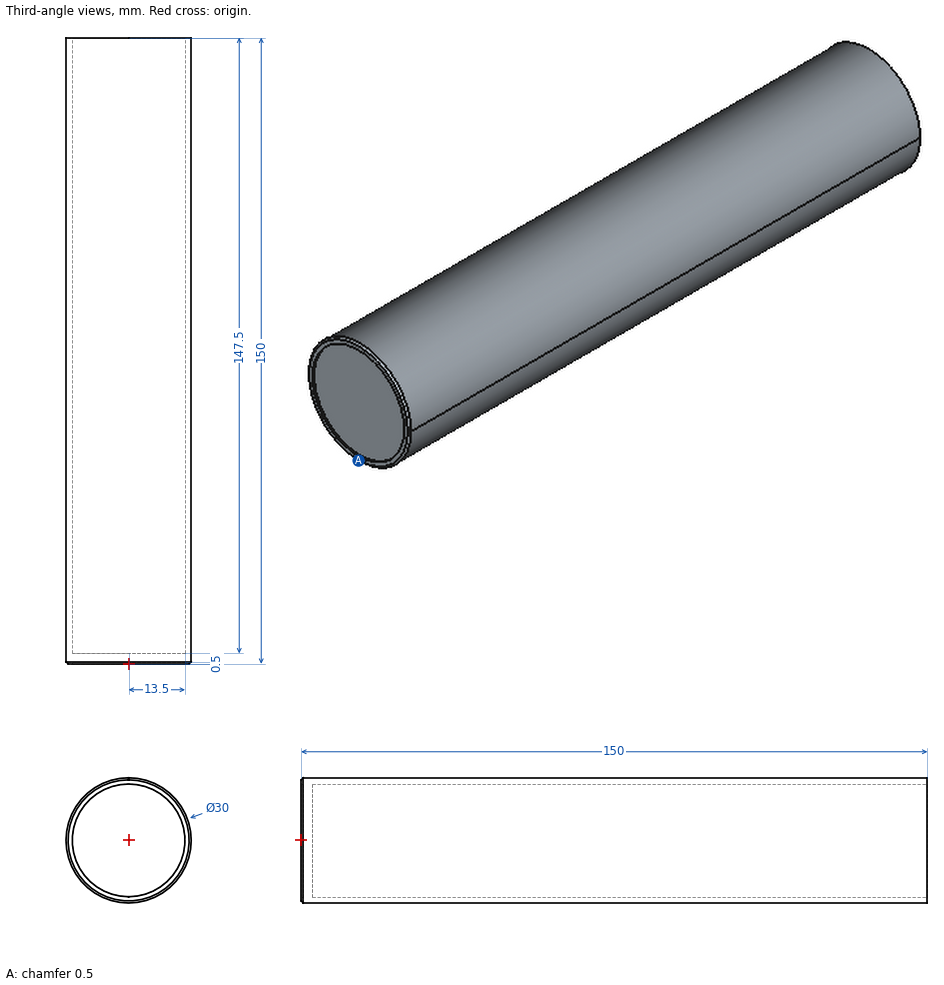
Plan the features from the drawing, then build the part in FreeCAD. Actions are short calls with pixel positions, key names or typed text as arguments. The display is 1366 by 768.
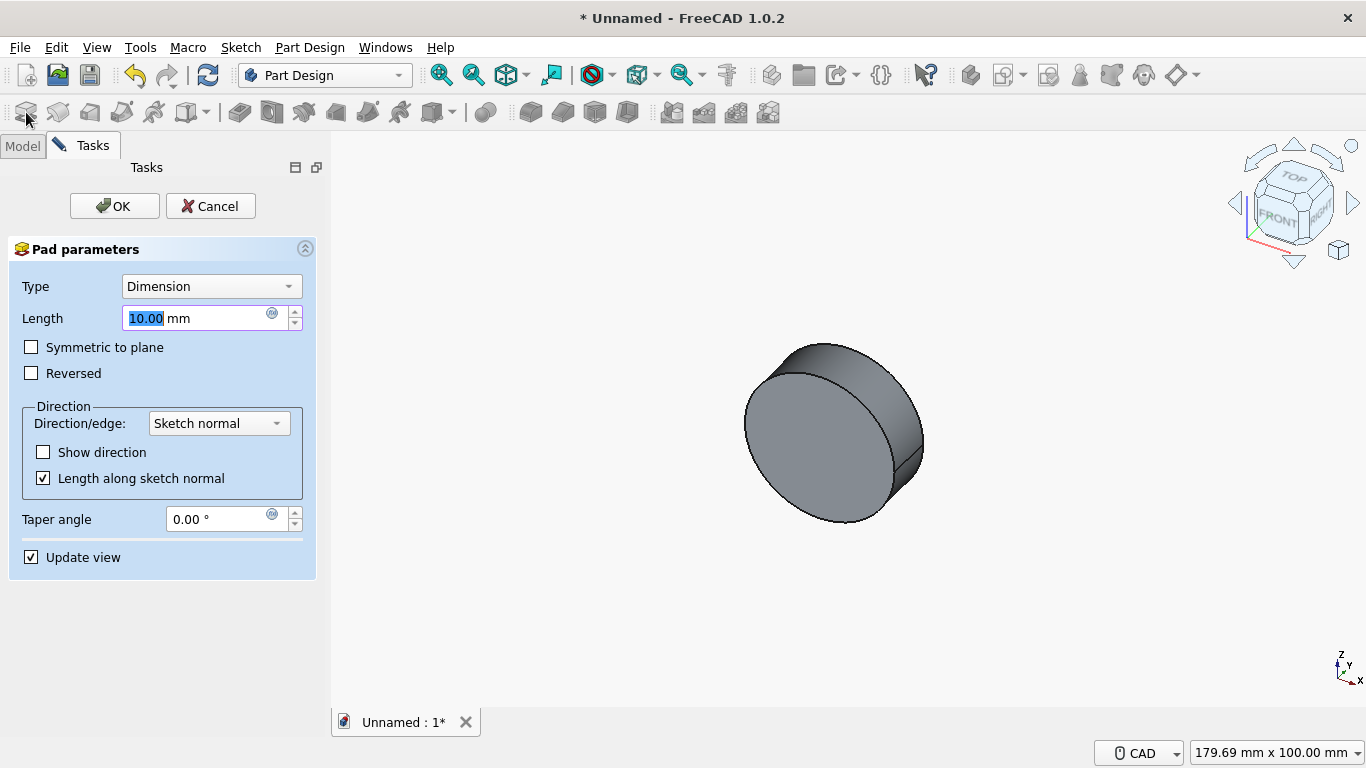
text(150)
key(Tab)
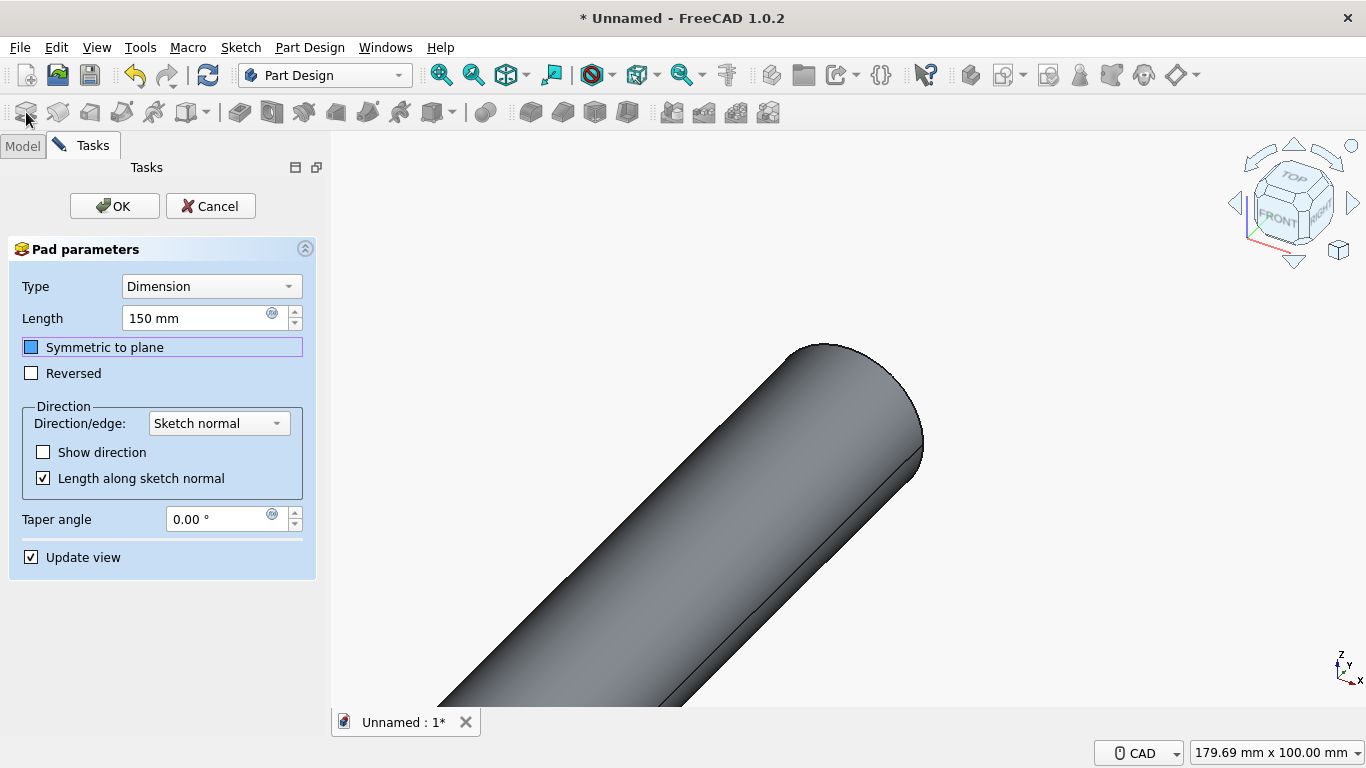
click(30, 373)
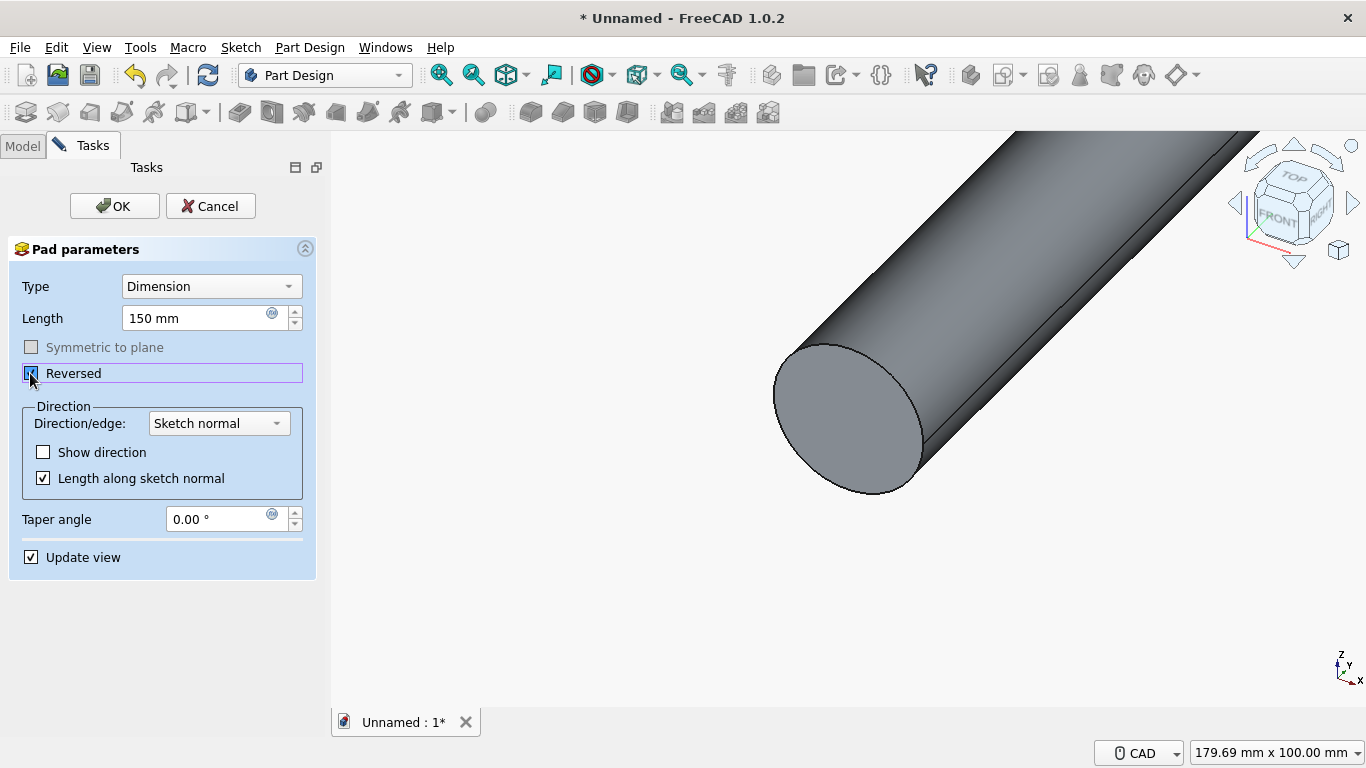
click(115, 206)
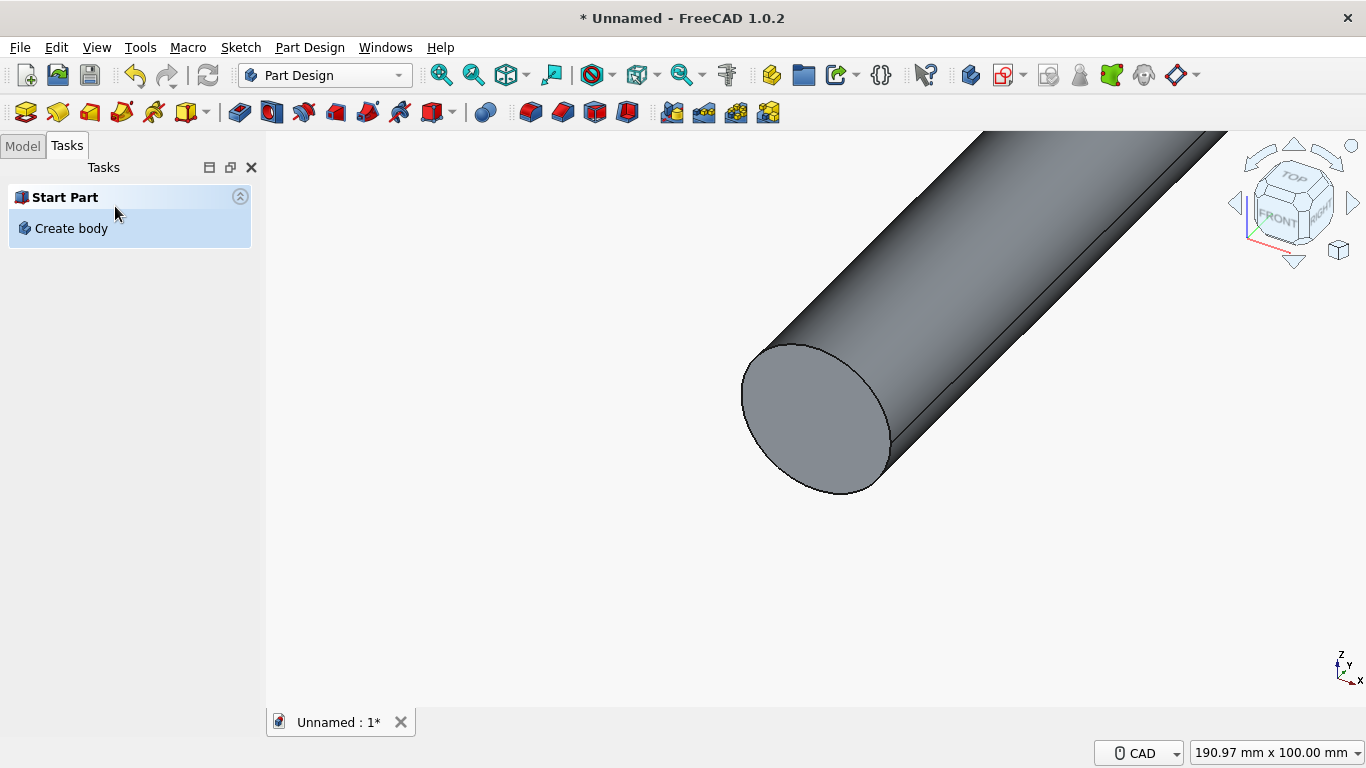
click(442, 76)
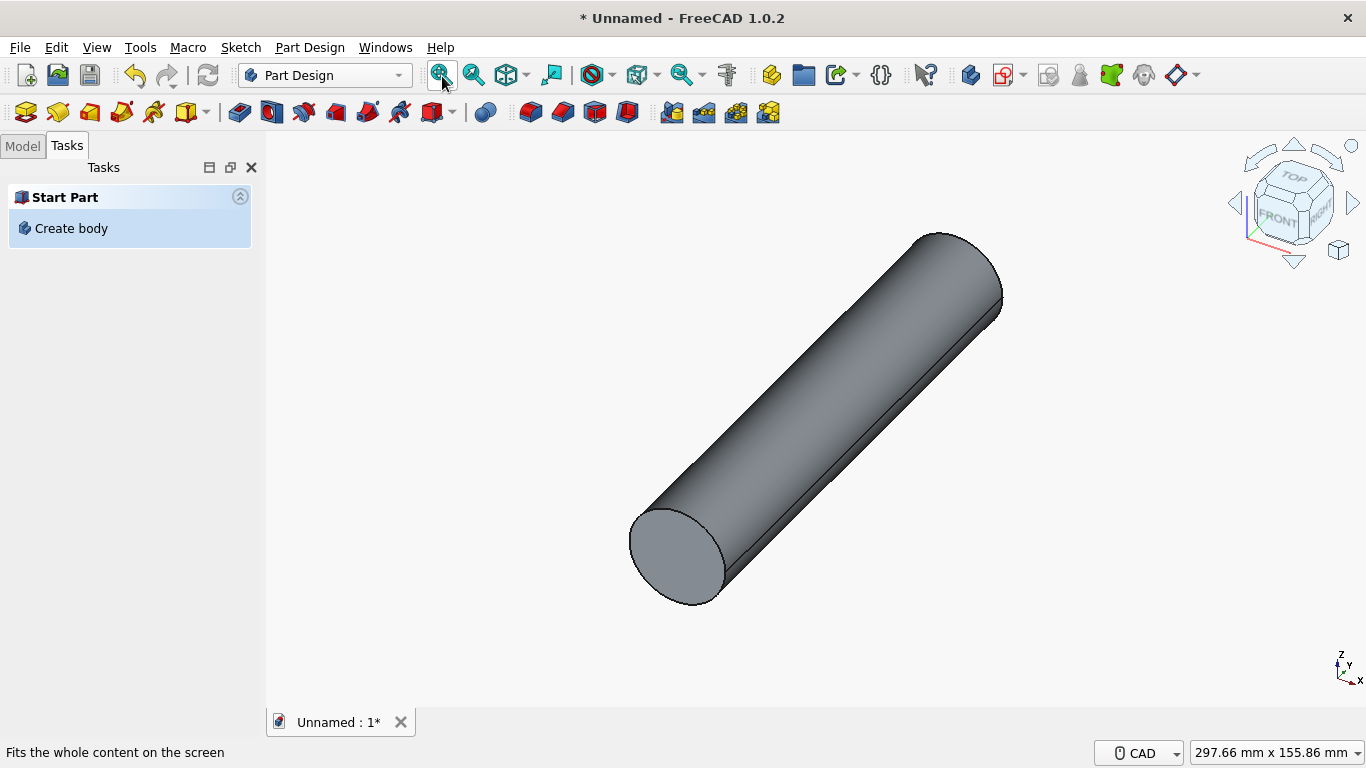
click(1004, 76)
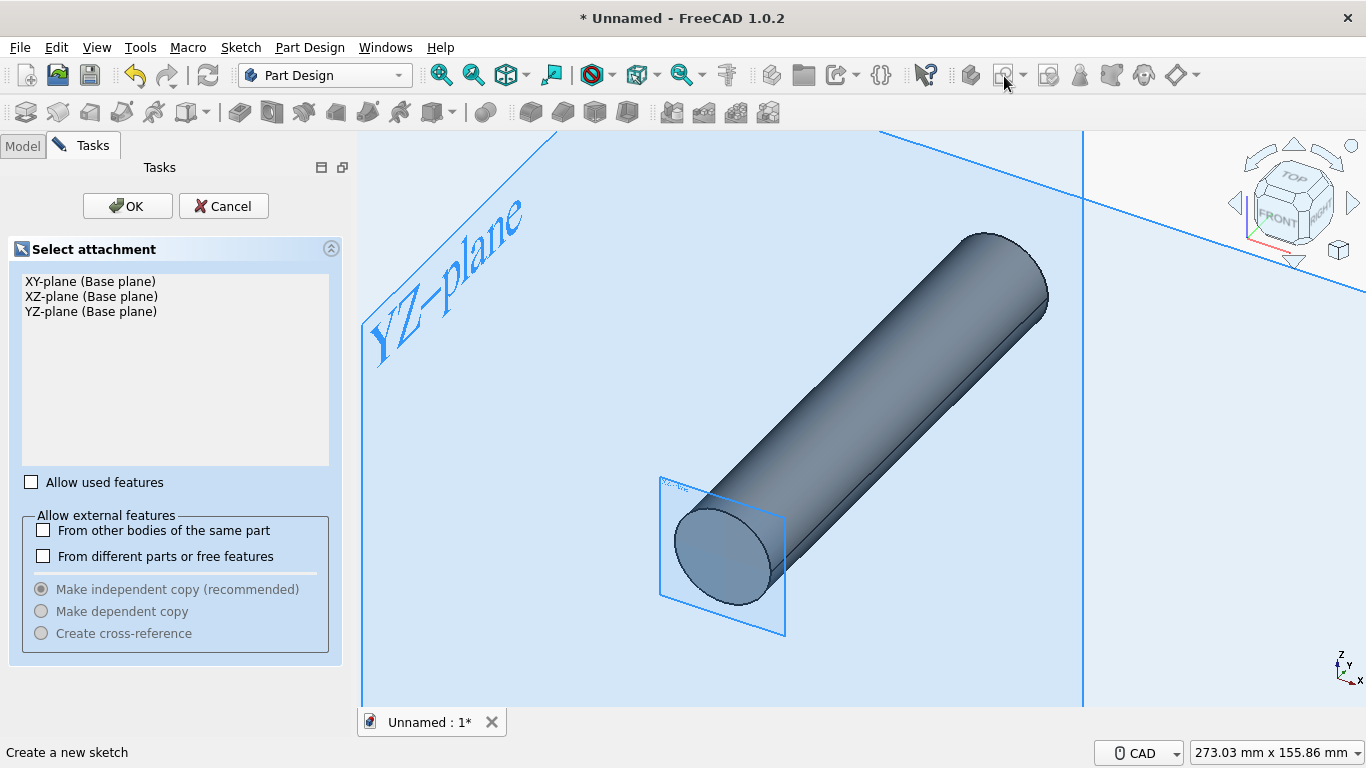
click(82, 282)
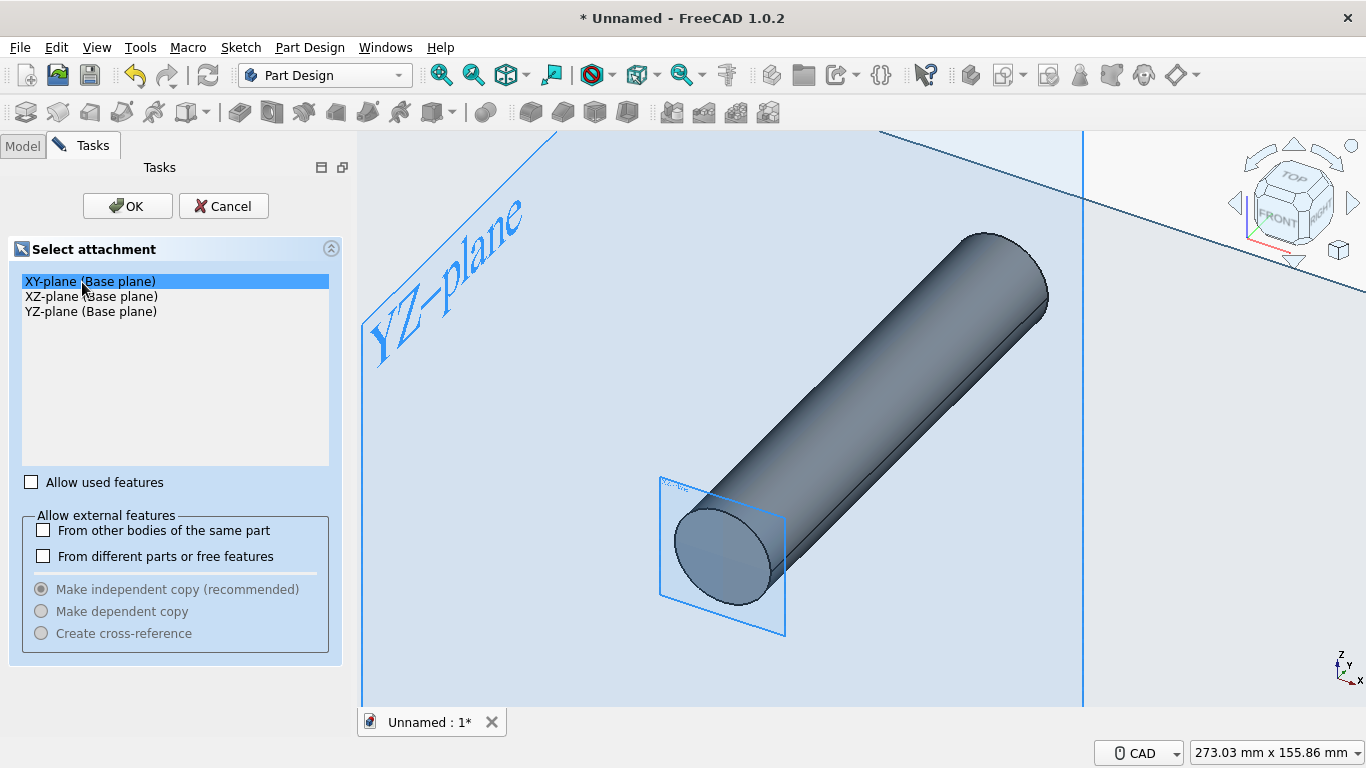
click(128, 206)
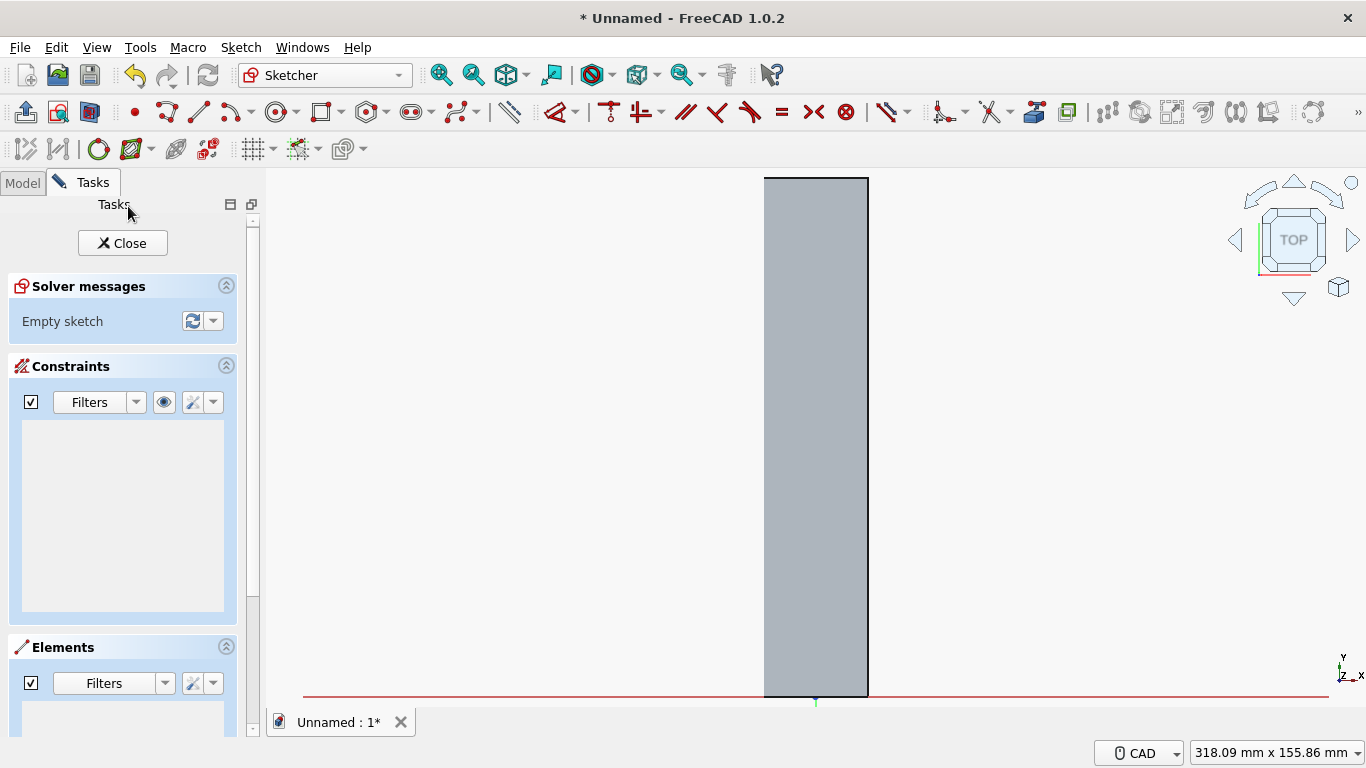
click(90, 112)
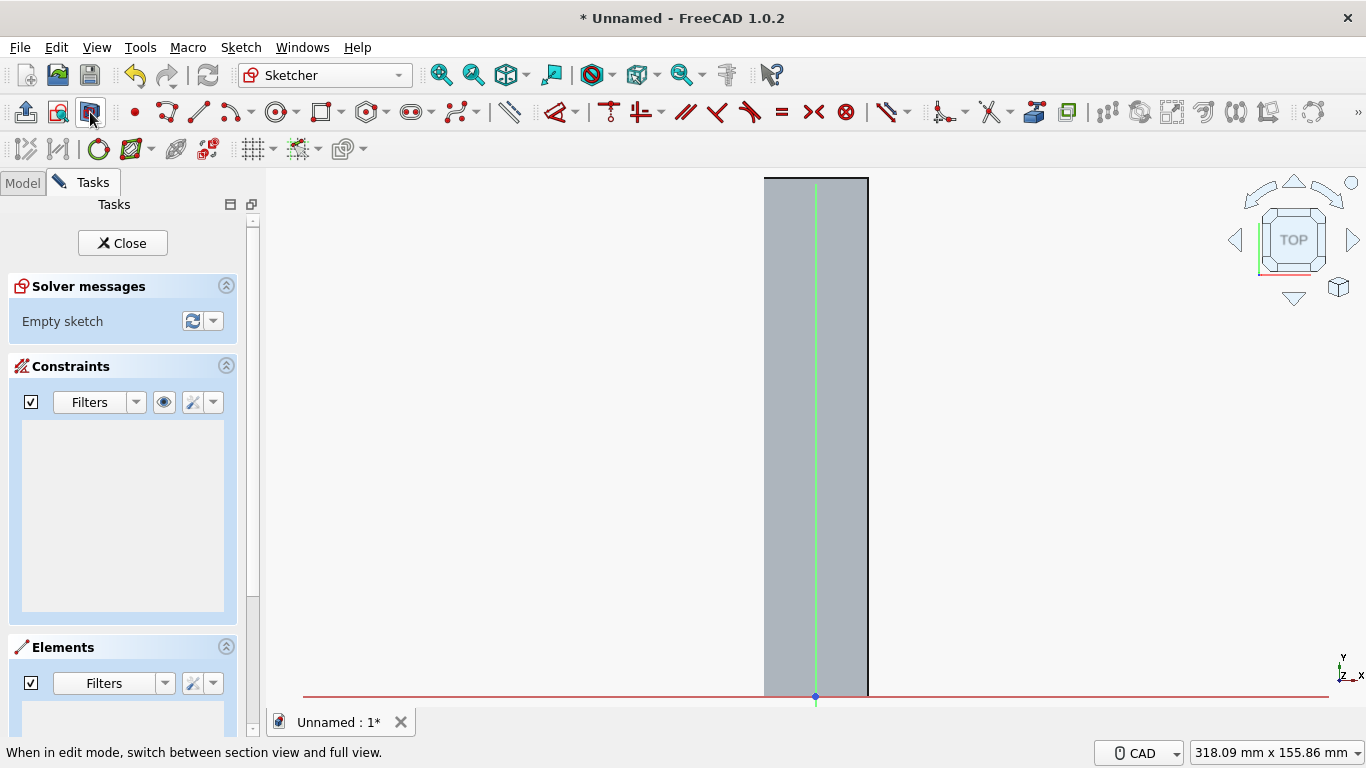
scroll(561, 437, down, 2)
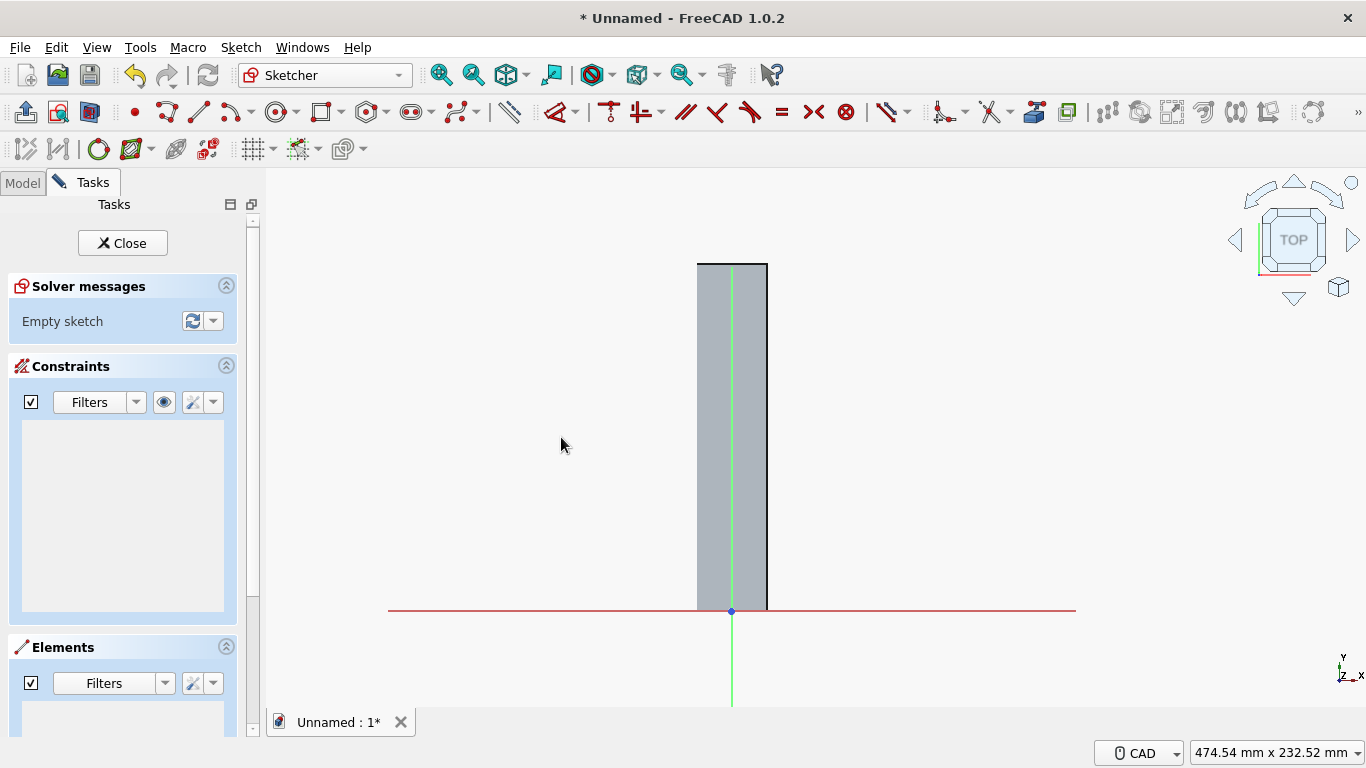
click(322, 112)